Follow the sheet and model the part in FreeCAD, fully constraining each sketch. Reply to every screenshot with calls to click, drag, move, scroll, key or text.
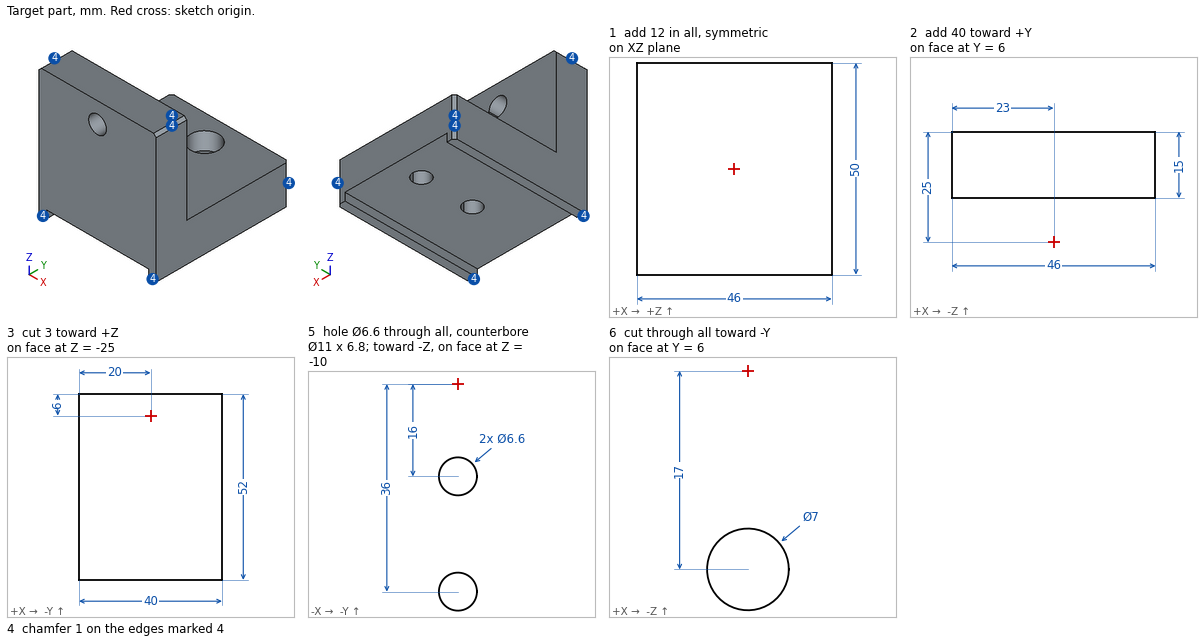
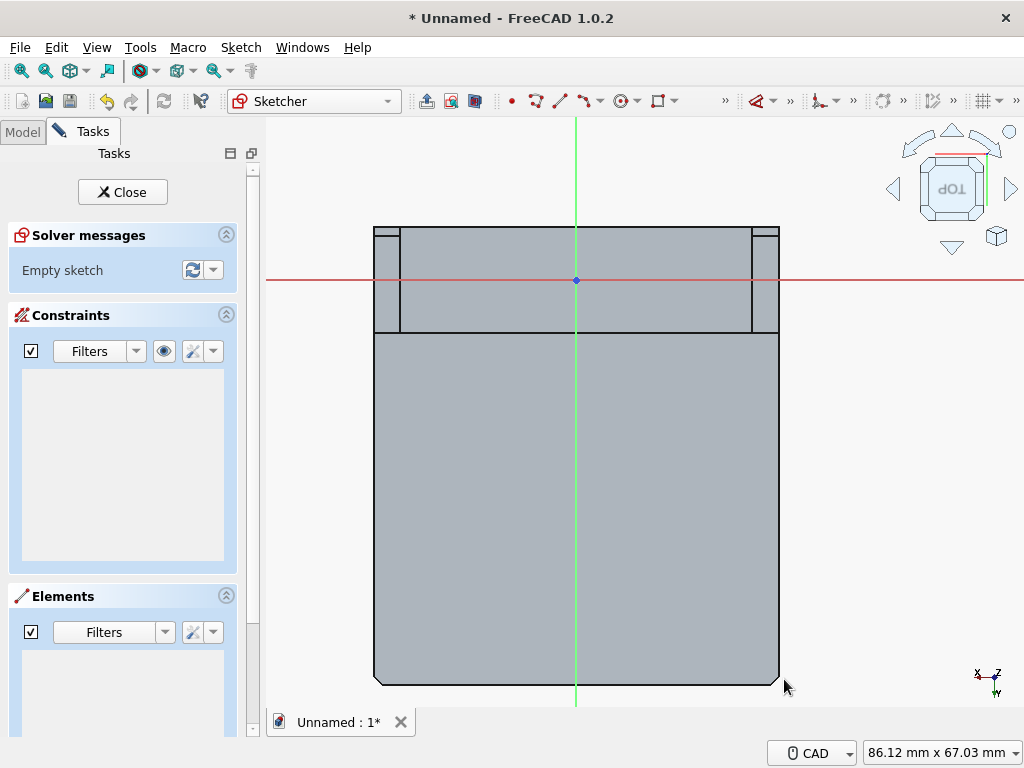
click(622, 102)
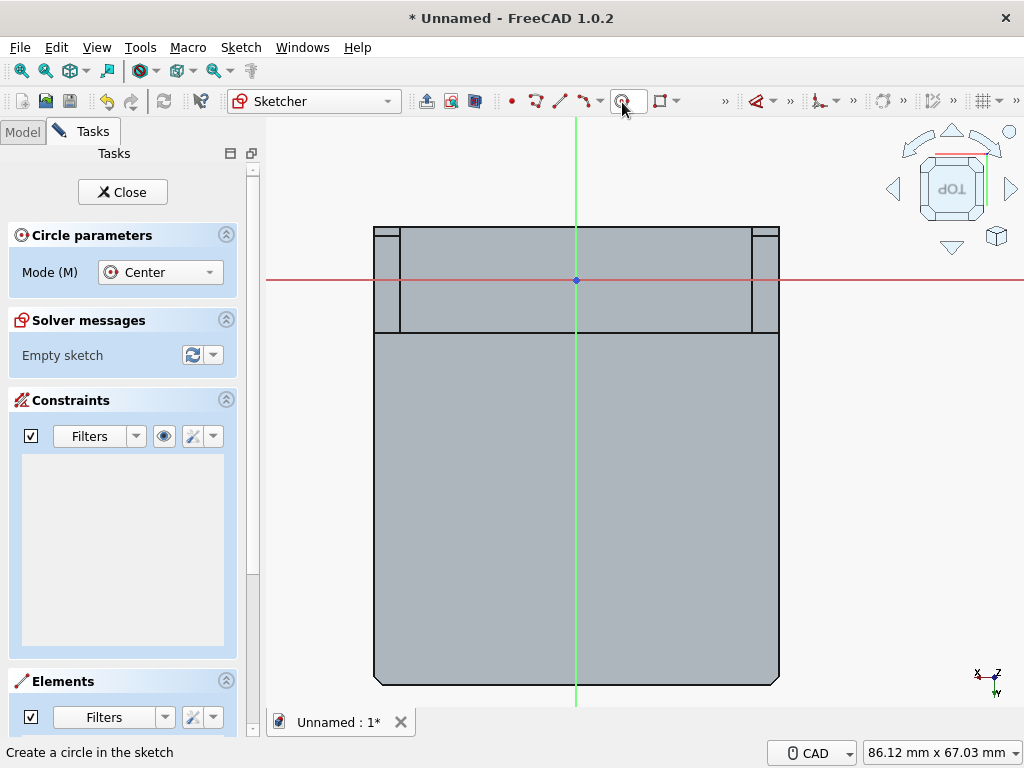
click(576, 421)
move(597, 401)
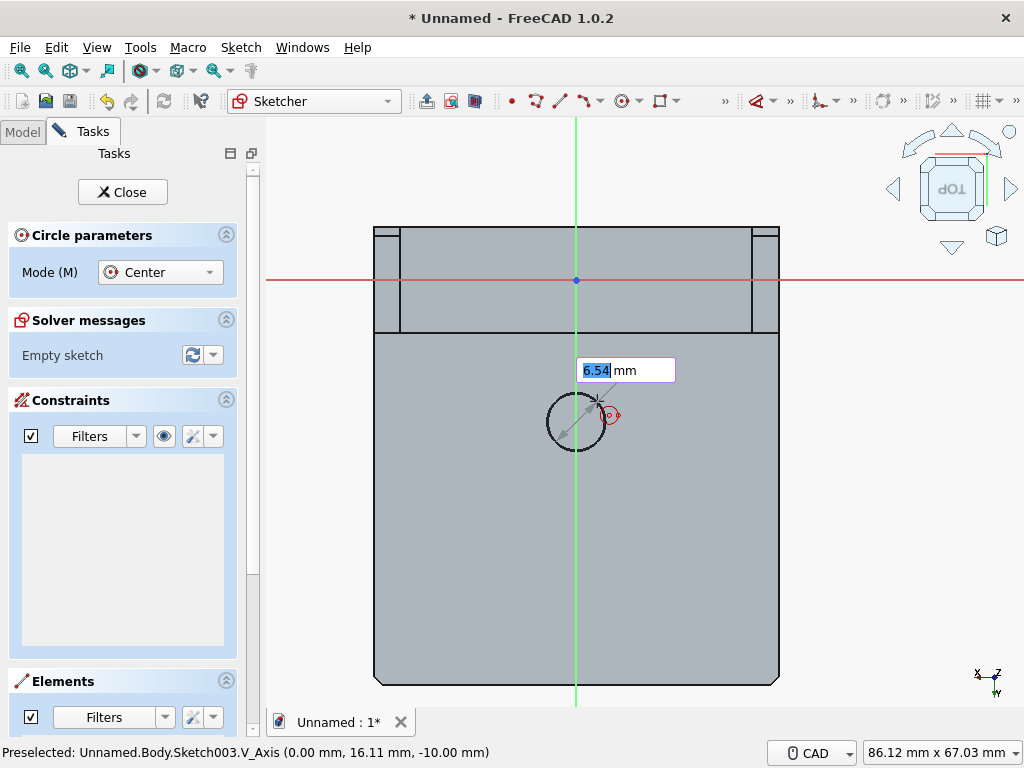
text(6.6)
key(Return)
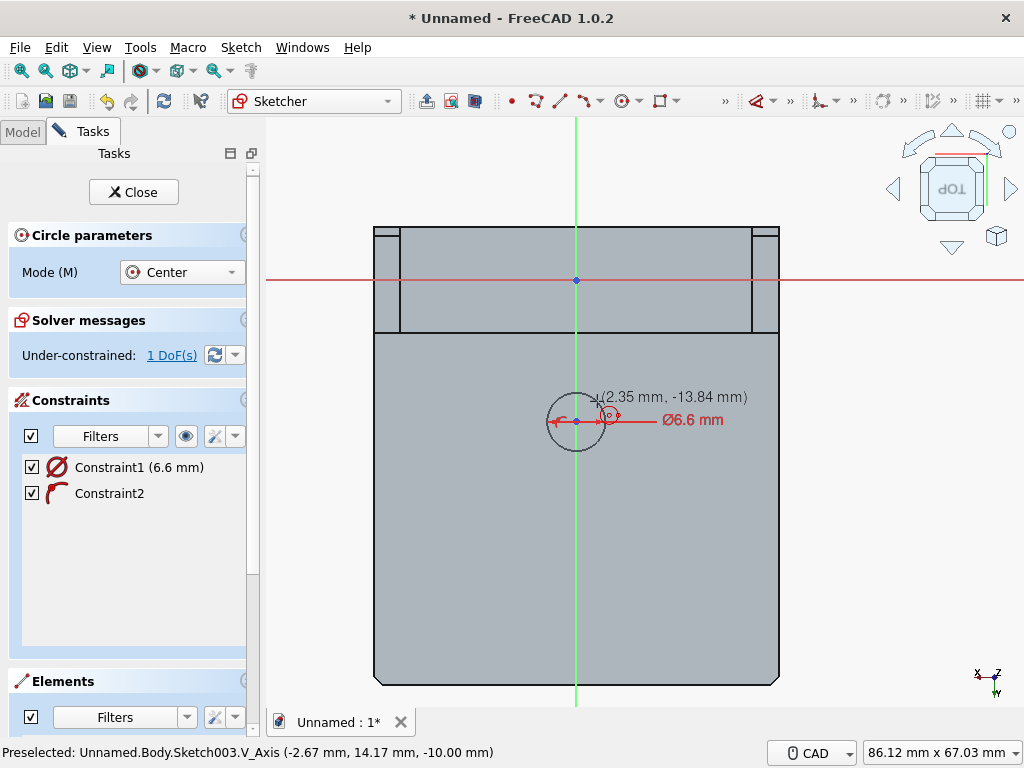
click(576, 597)
move(597, 577)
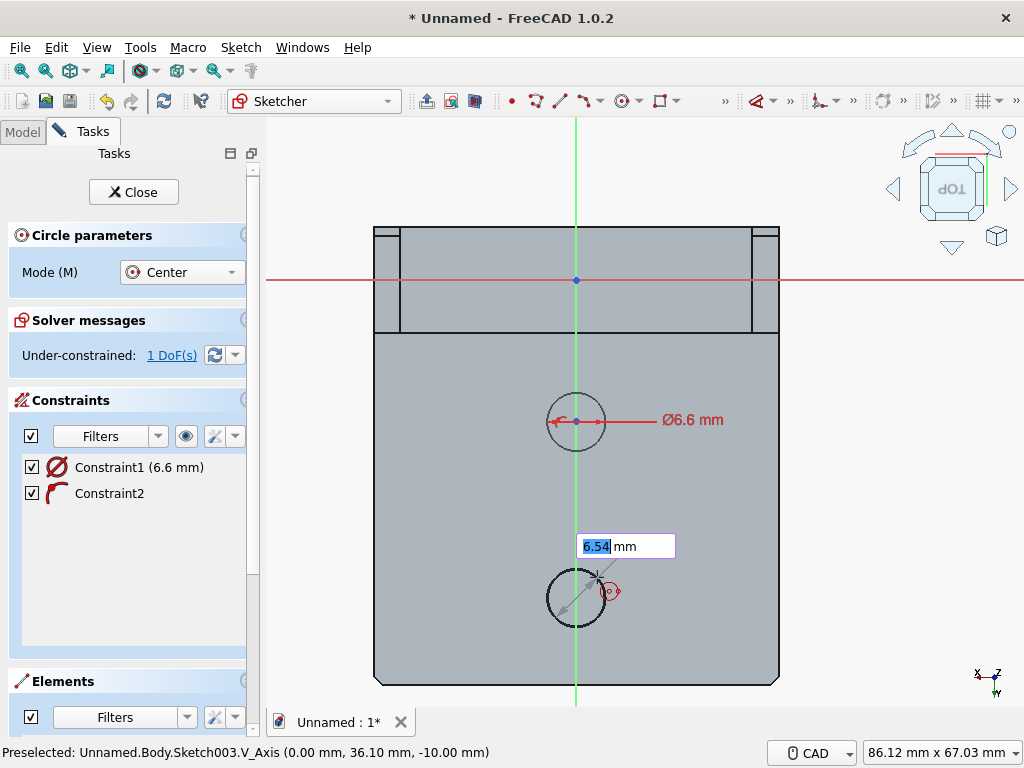
text(6.6)
key(Return)
key(Escape)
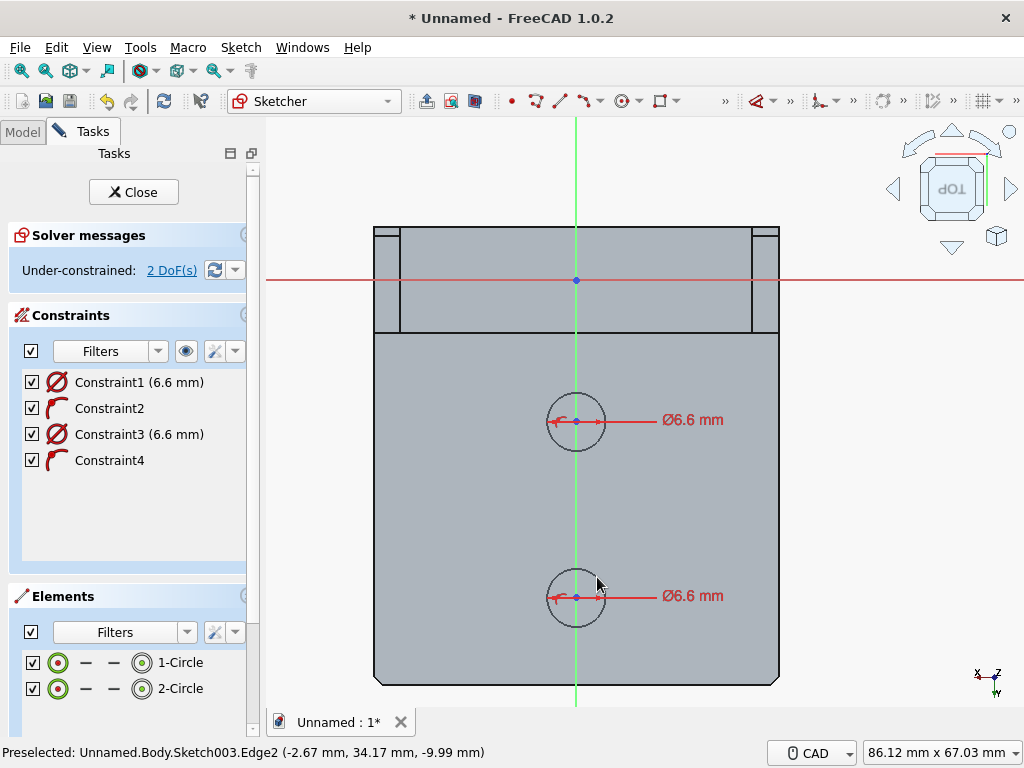
click(756, 102)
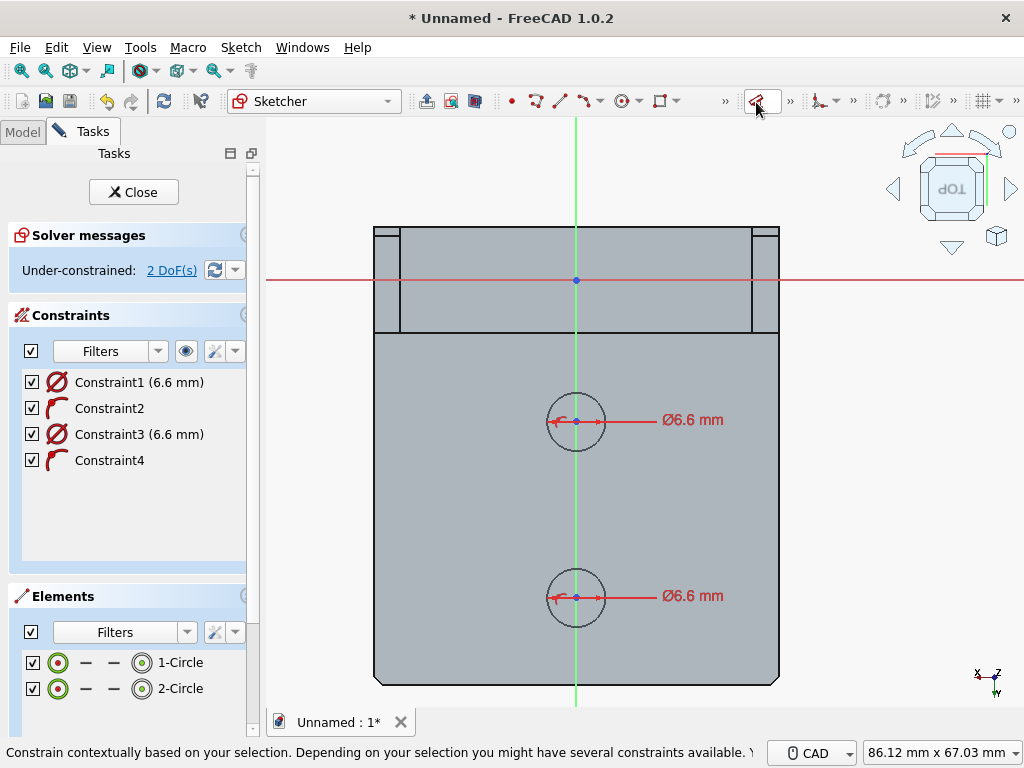
click(576, 422)
click(610, 351)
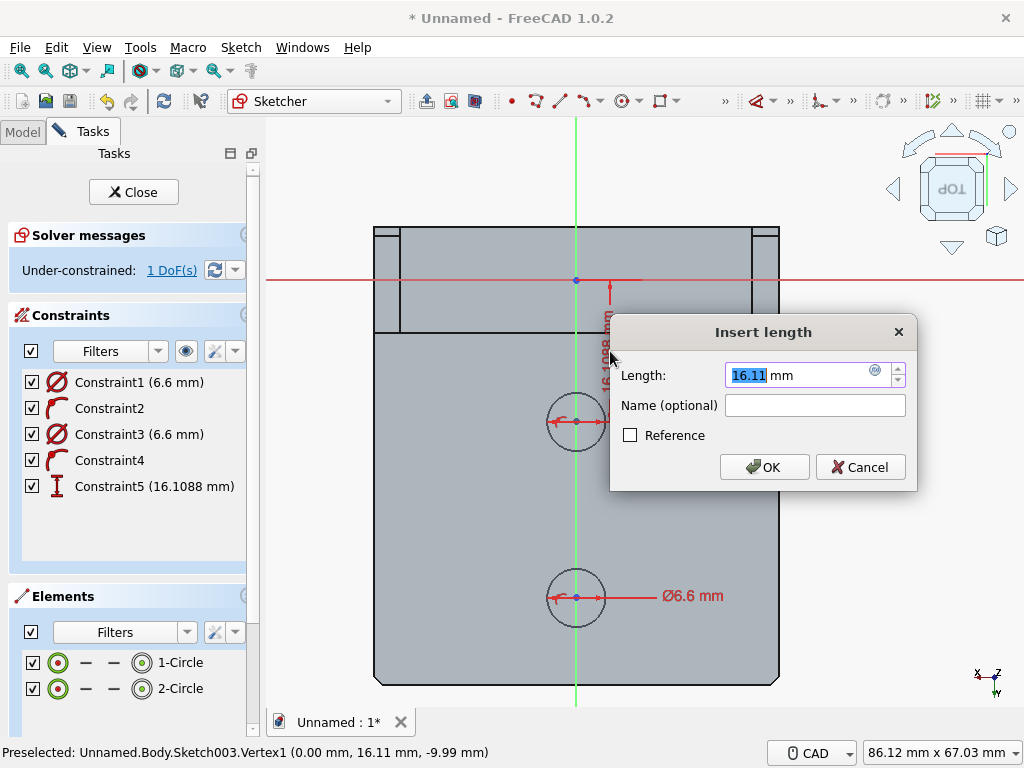
text(16)
key(Return)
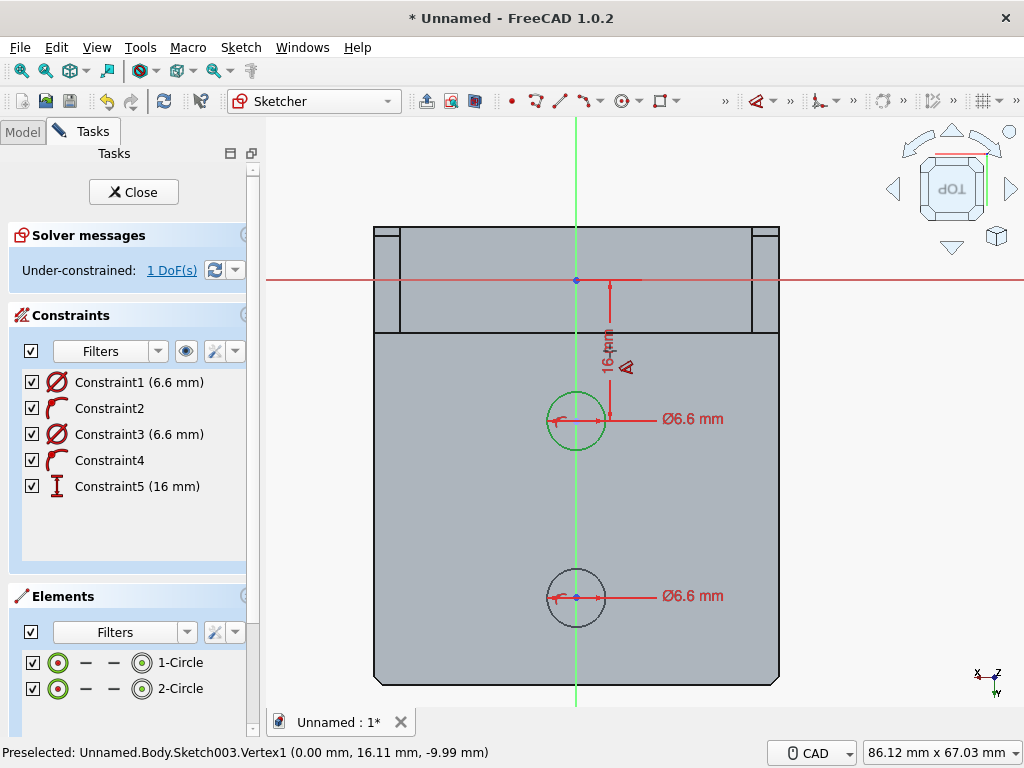
click(576, 598)
click(610, 512)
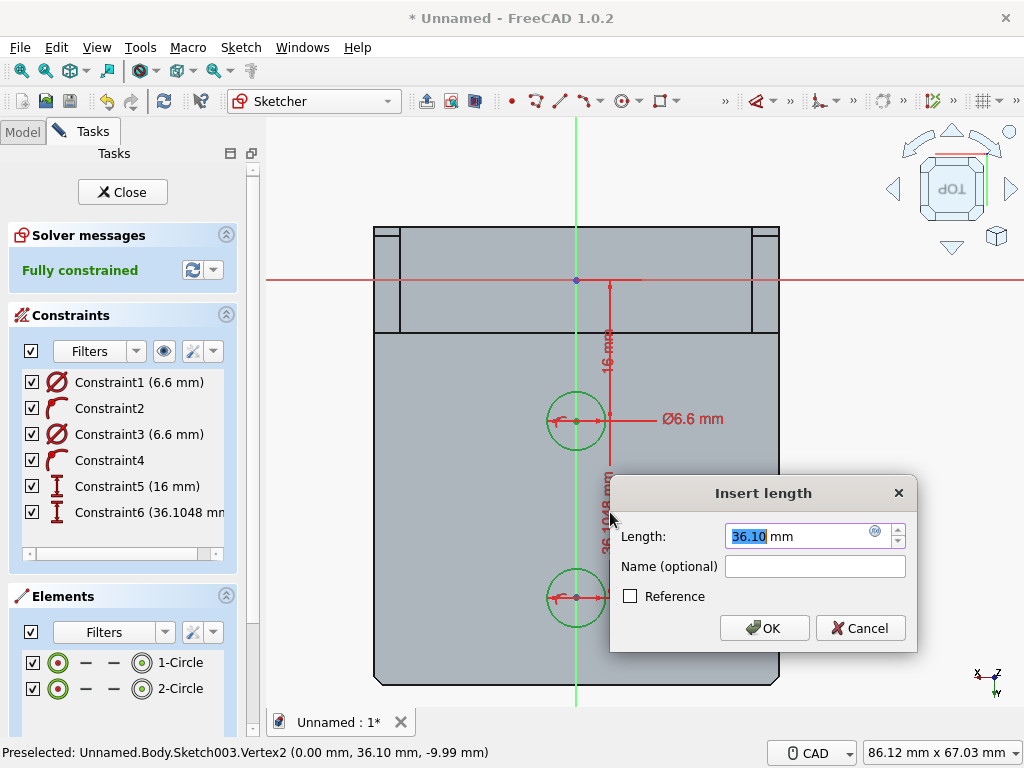
text(36)
key(Return)
key(Escape)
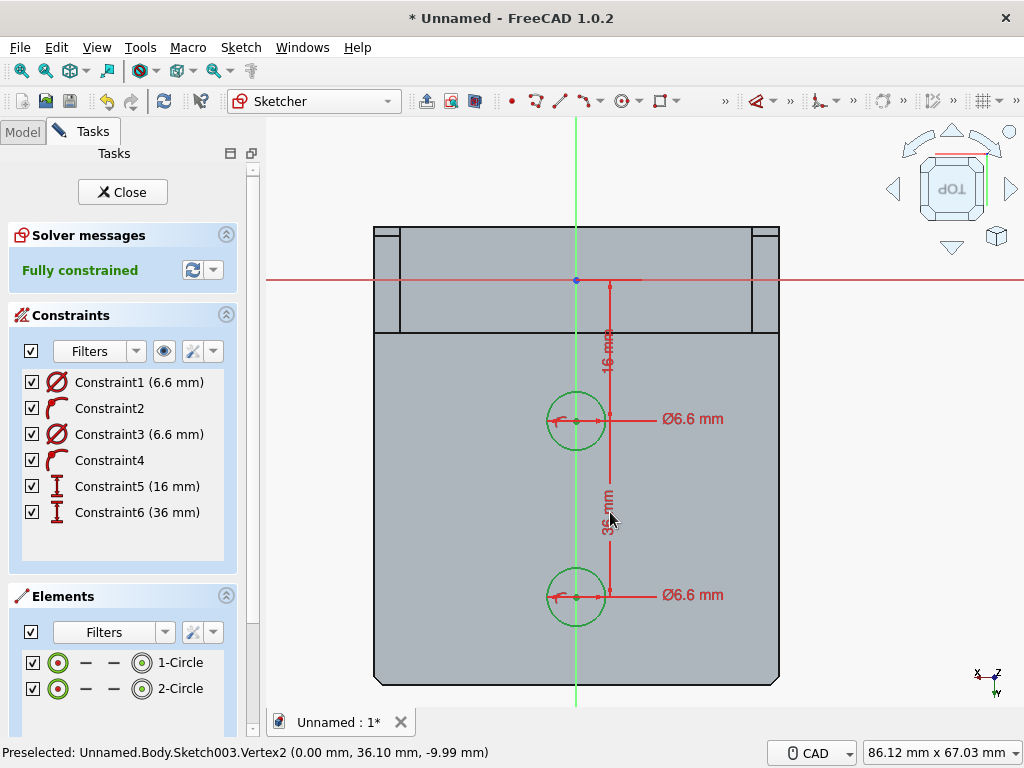
click(123, 192)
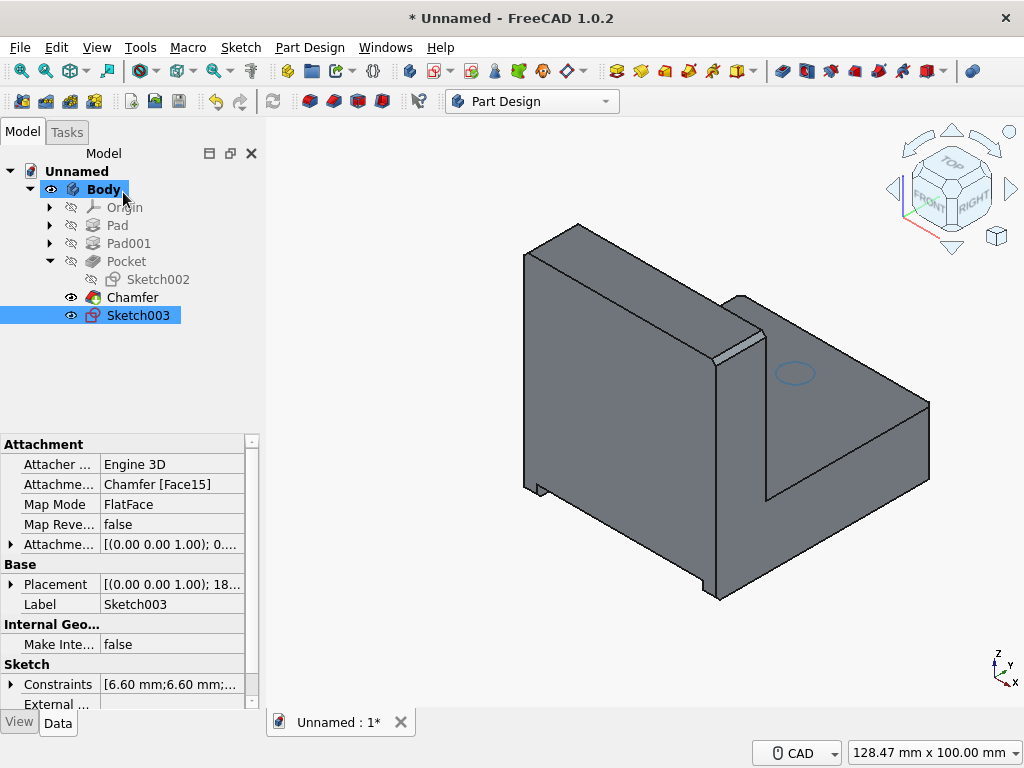
click(808, 72)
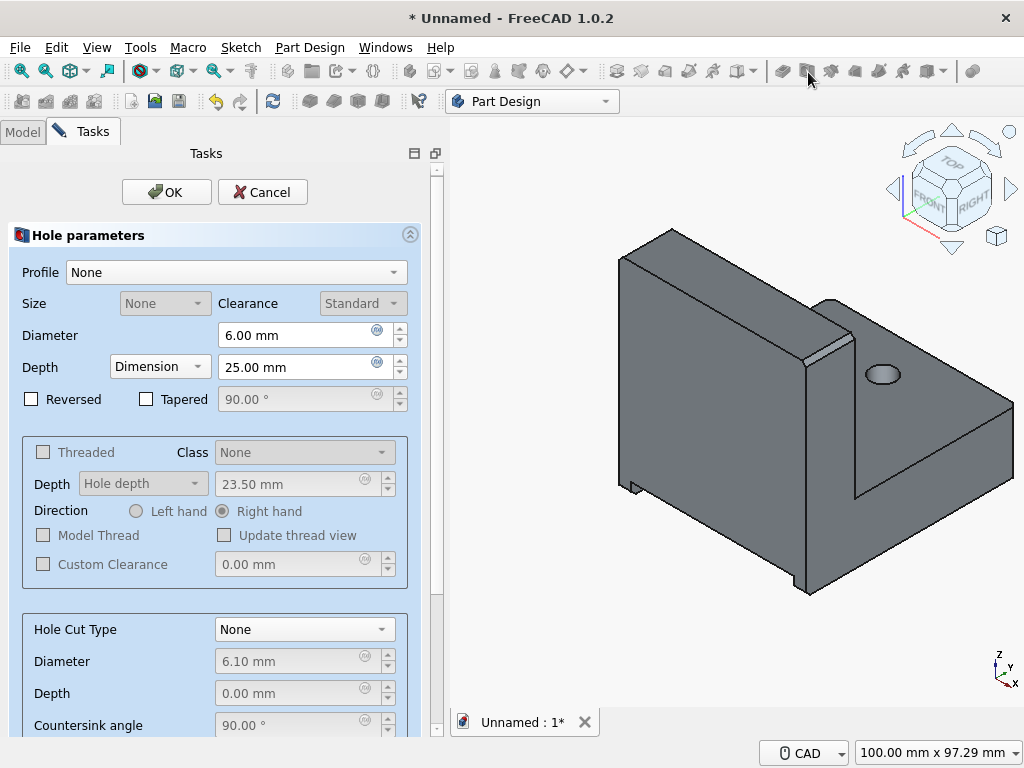
triple_click(305, 335)